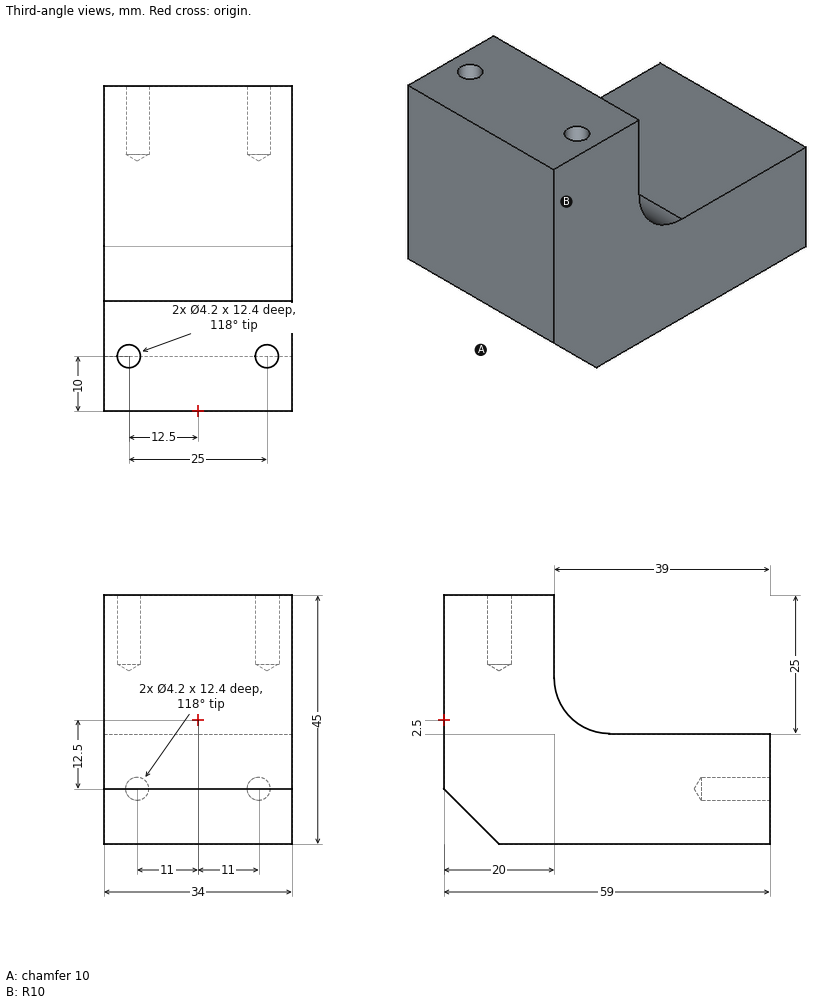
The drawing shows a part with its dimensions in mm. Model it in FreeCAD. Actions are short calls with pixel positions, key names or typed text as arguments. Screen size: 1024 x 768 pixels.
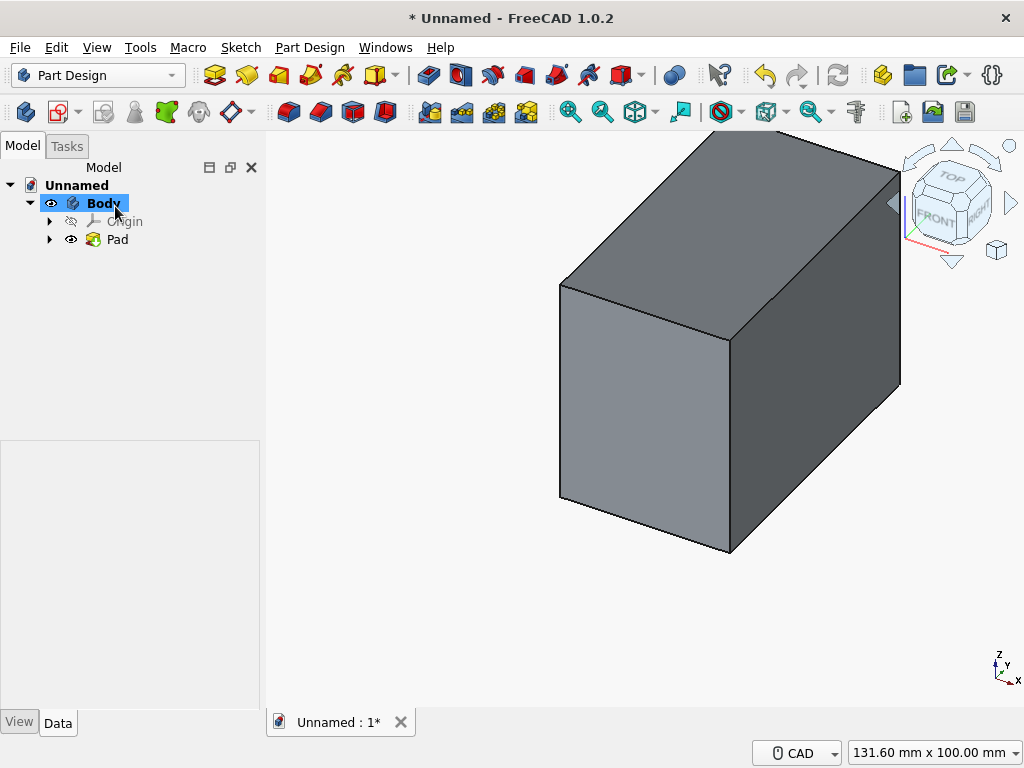
click(572, 112)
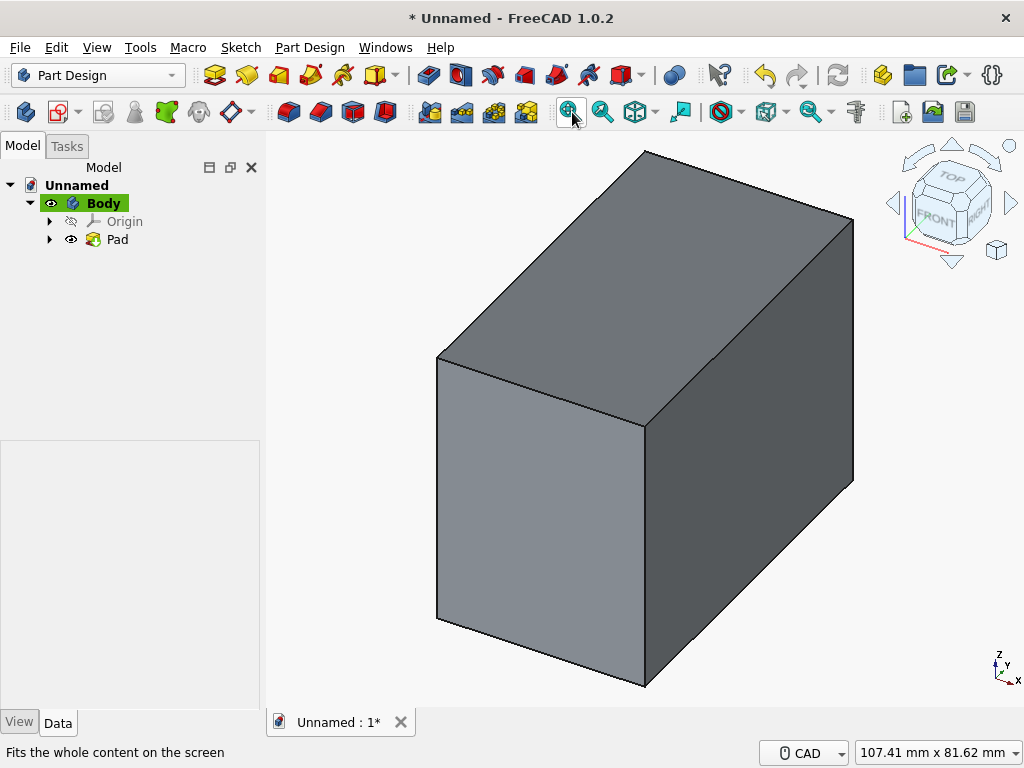
click(749, 452)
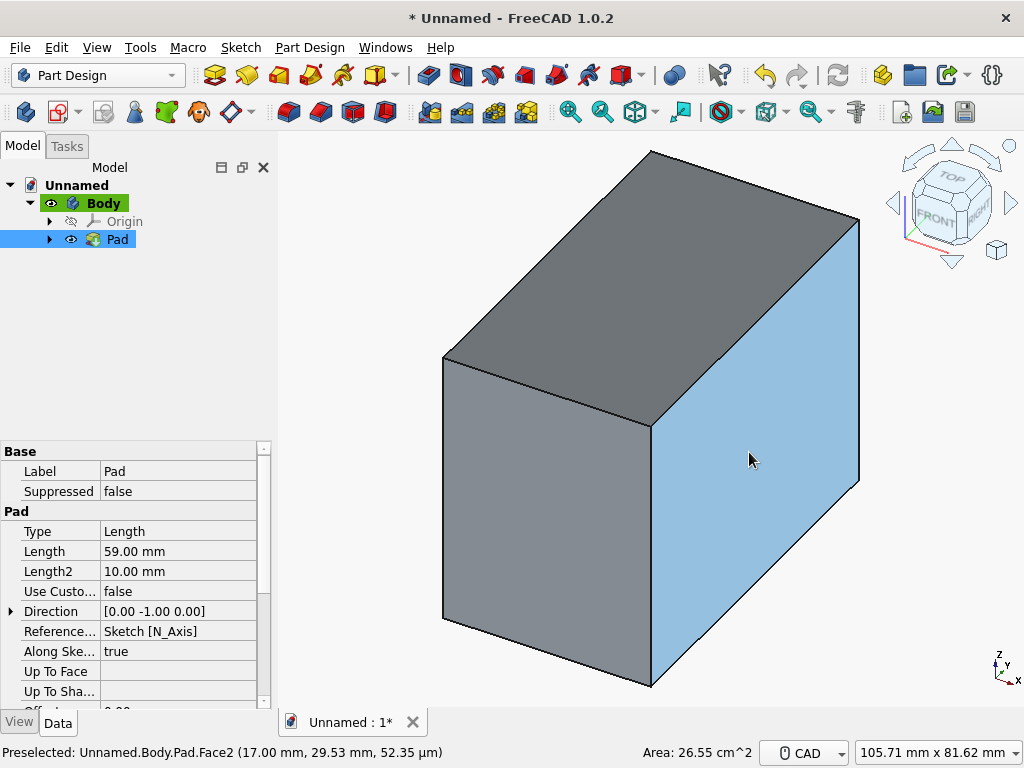
click(58, 112)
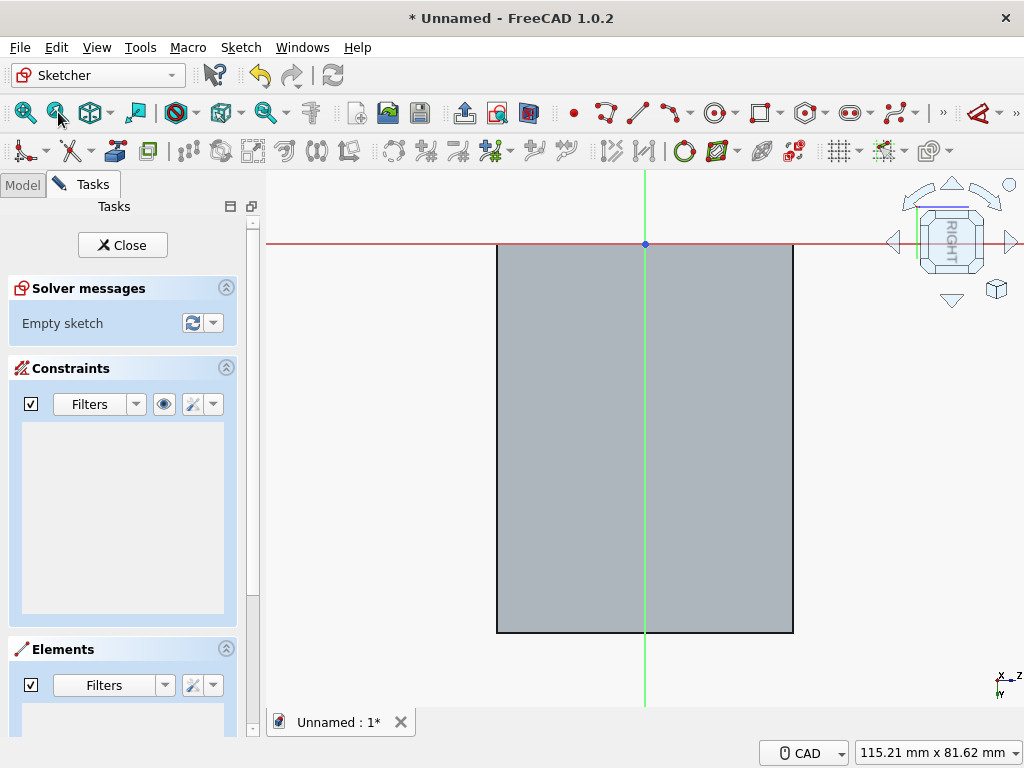
click(760, 114)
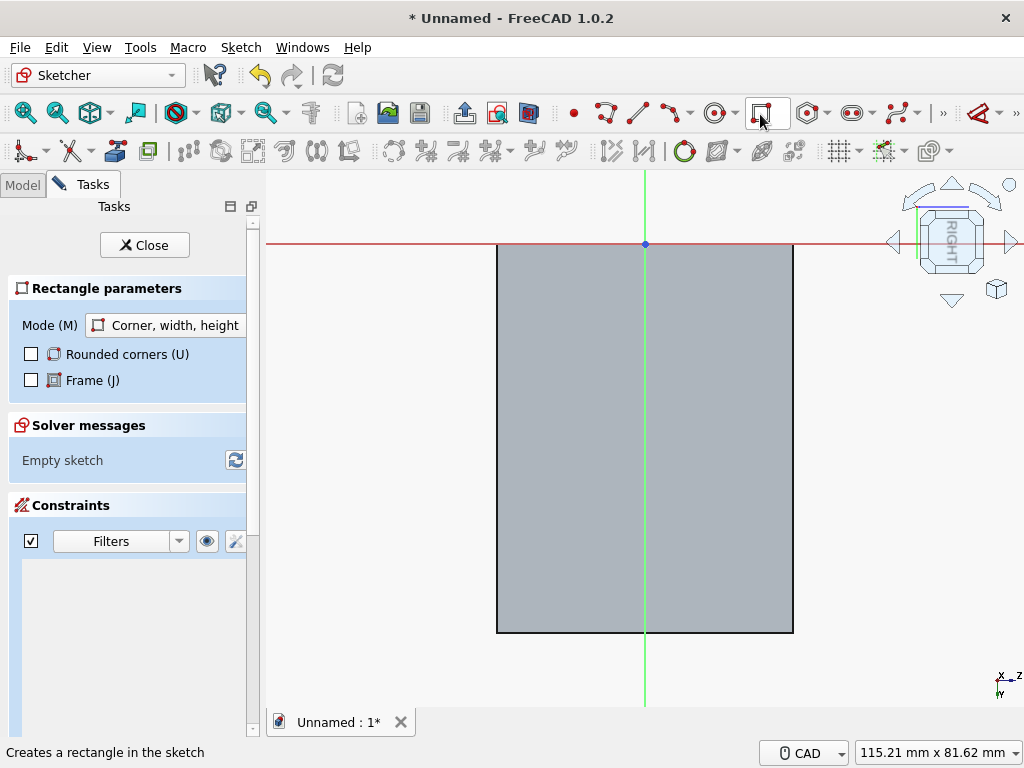
click(629, 376)
move(793, 633)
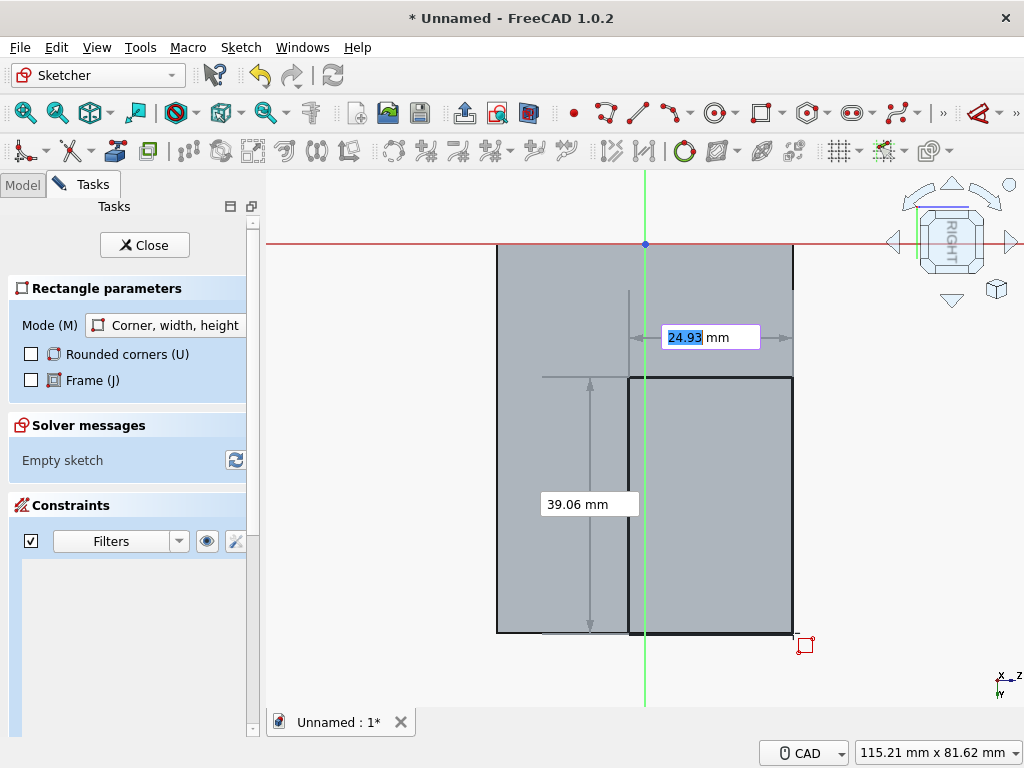
text(25)
key(Tab)
text(39)
key(Return)
key(Escape)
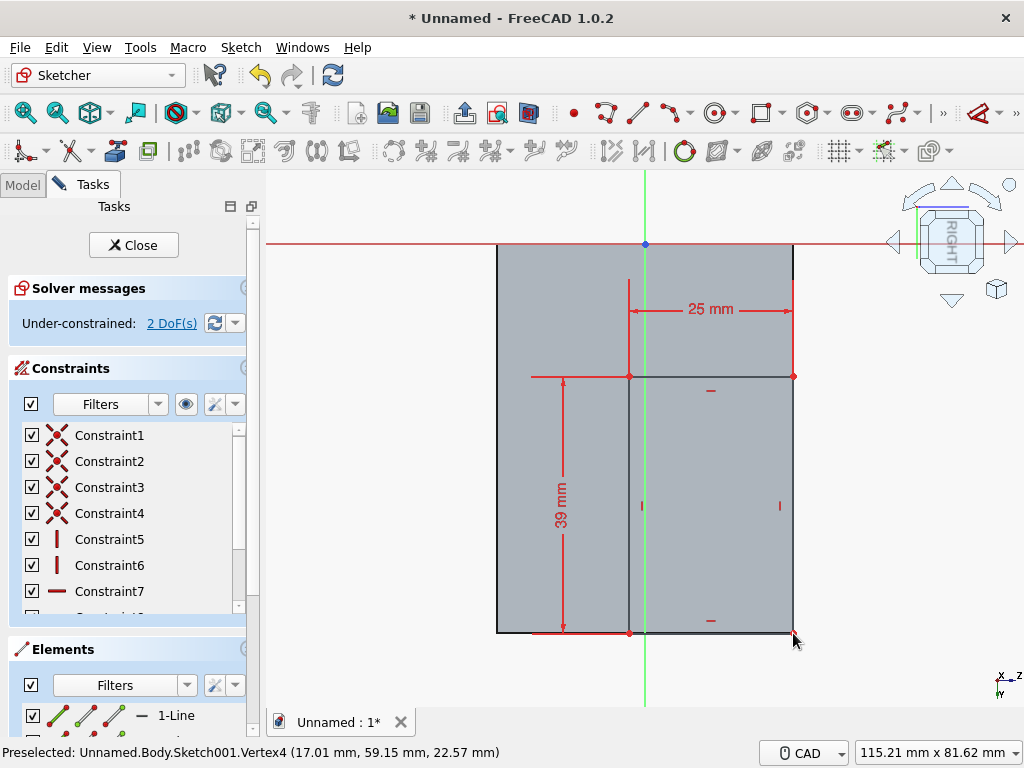
click(629, 377)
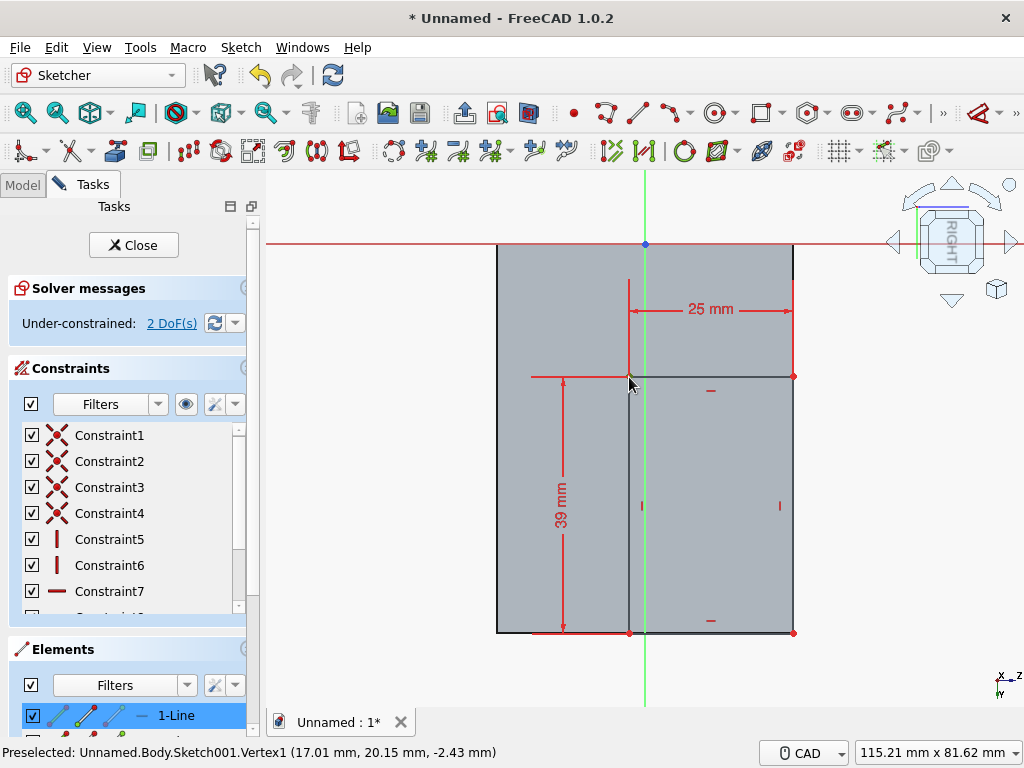
click(1002, 114)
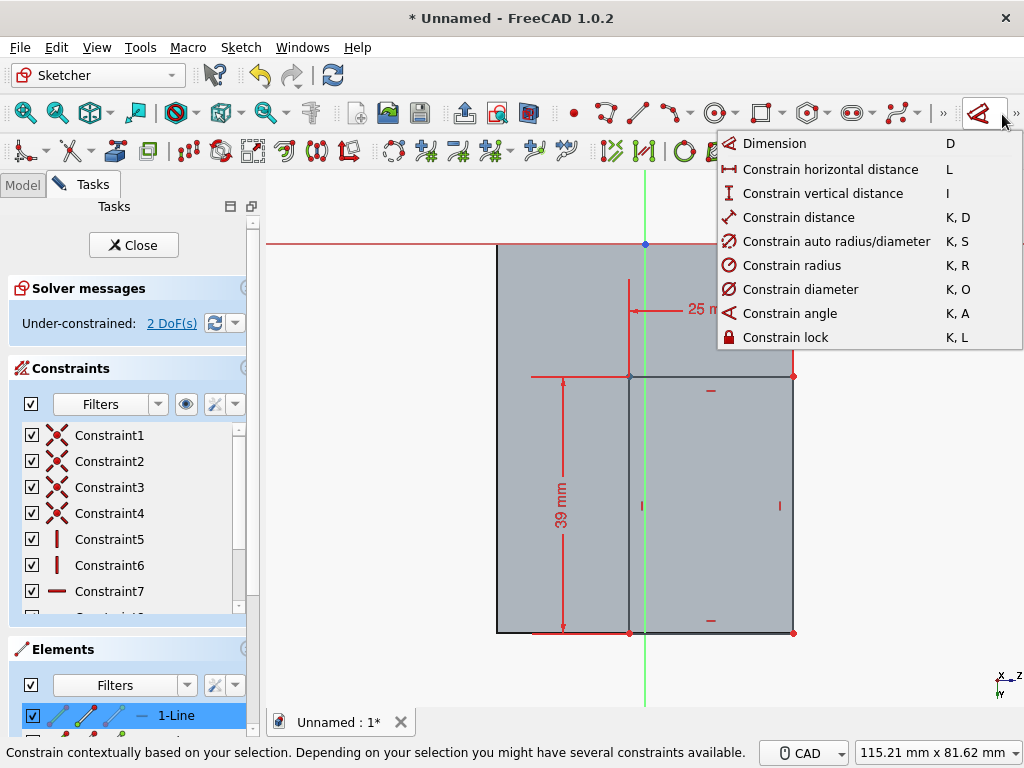
click(870, 193)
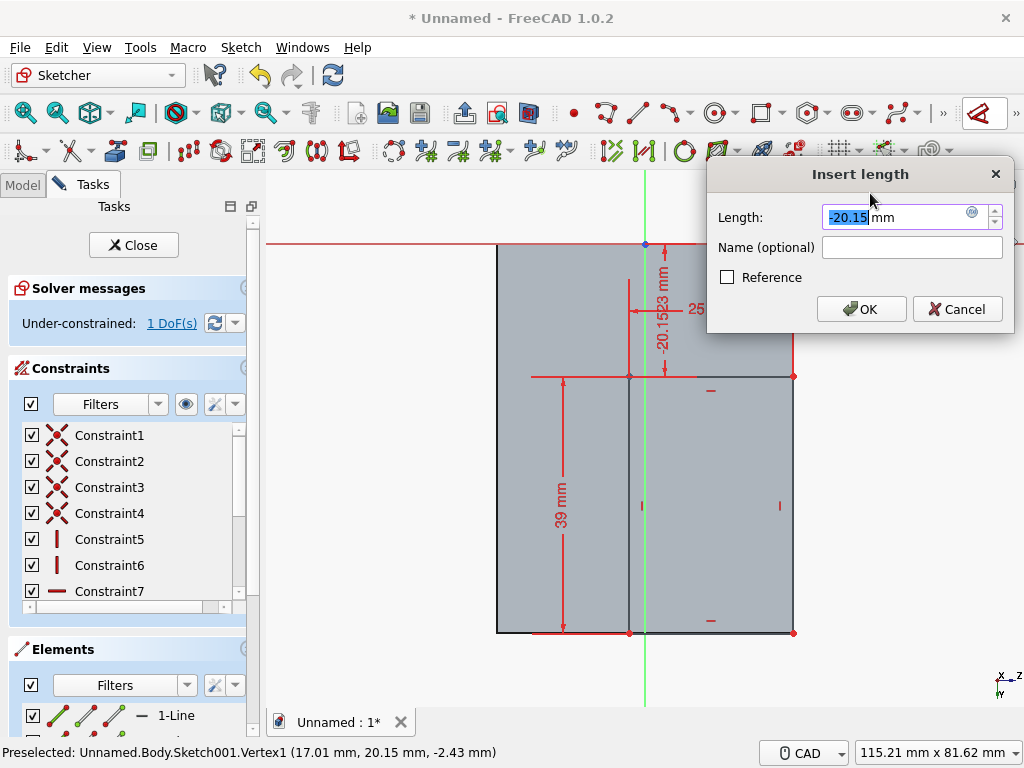
text(-20)
key(Return)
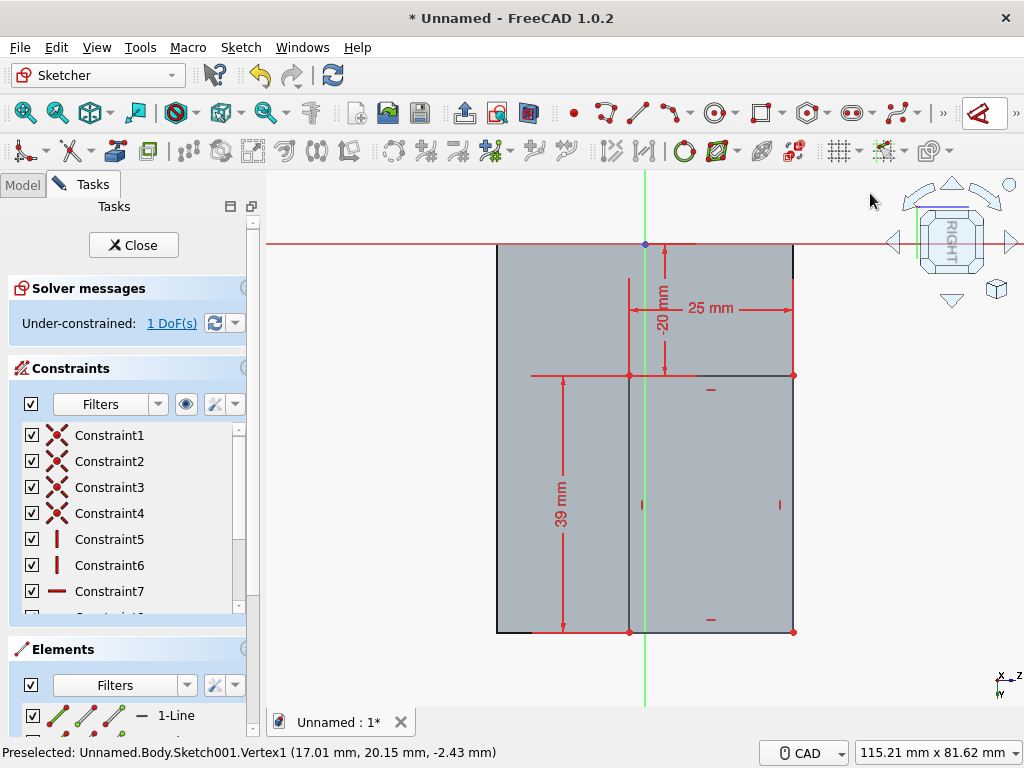
scroll(629, 376, up, 5)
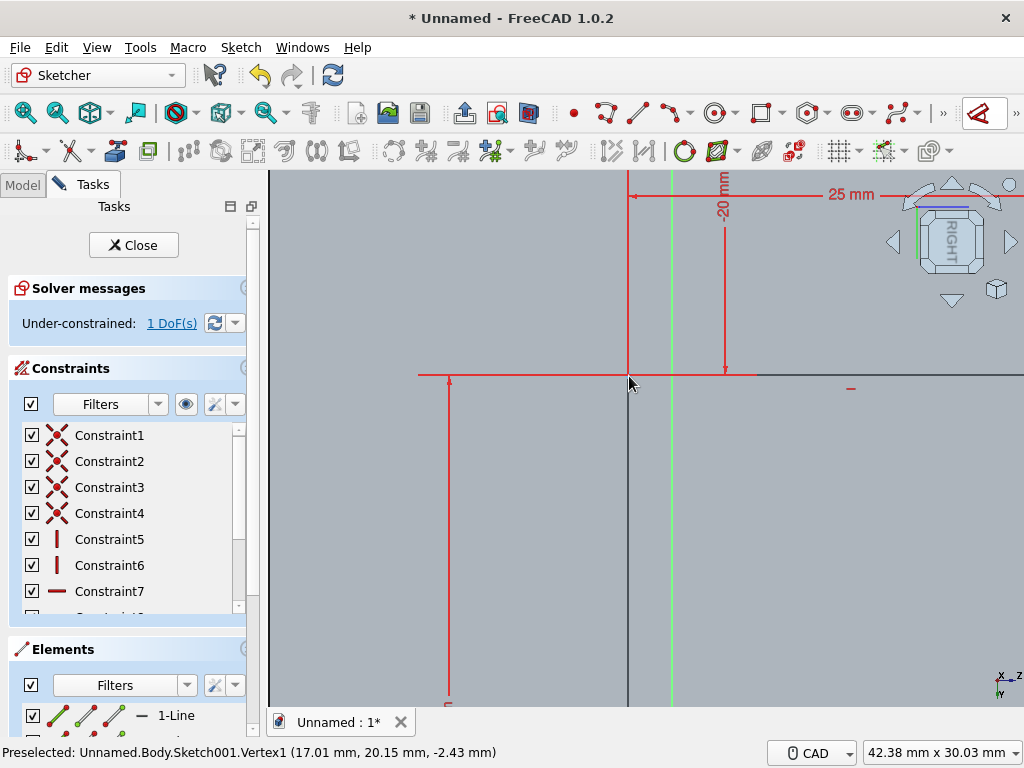
click(628, 375)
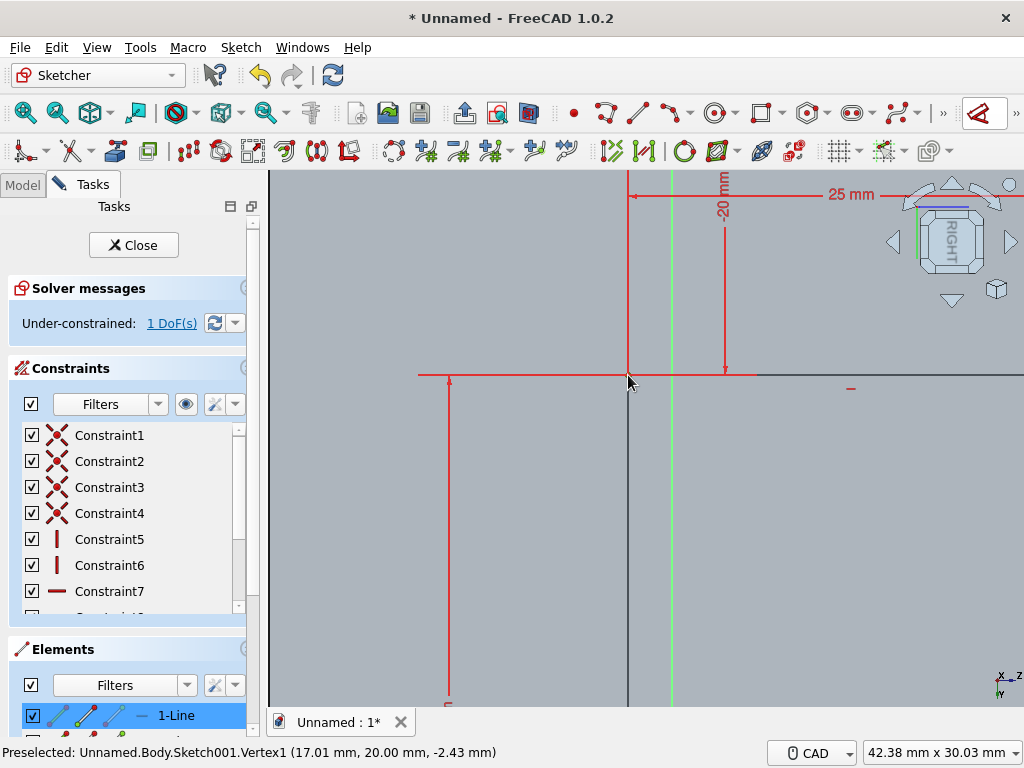
key(l)